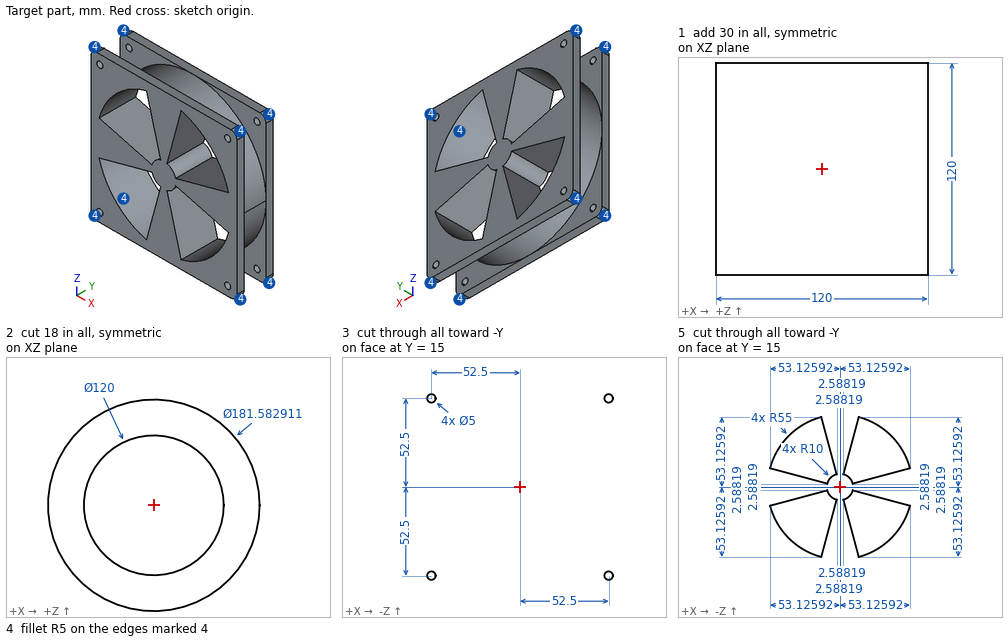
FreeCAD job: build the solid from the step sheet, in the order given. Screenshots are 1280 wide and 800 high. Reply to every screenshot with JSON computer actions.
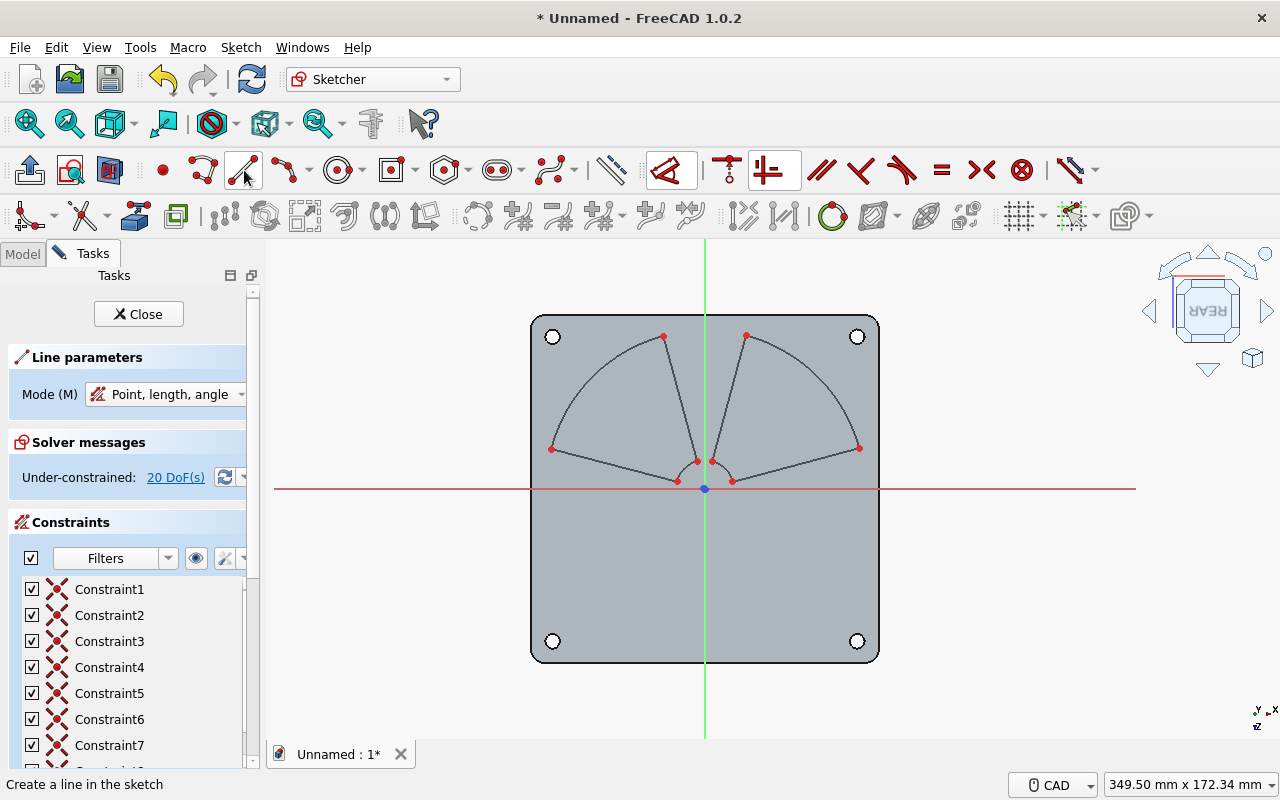
{"action": "scroll", "coordinate": [712, 517], "scroll_direction": "up", "scroll_amount": 4}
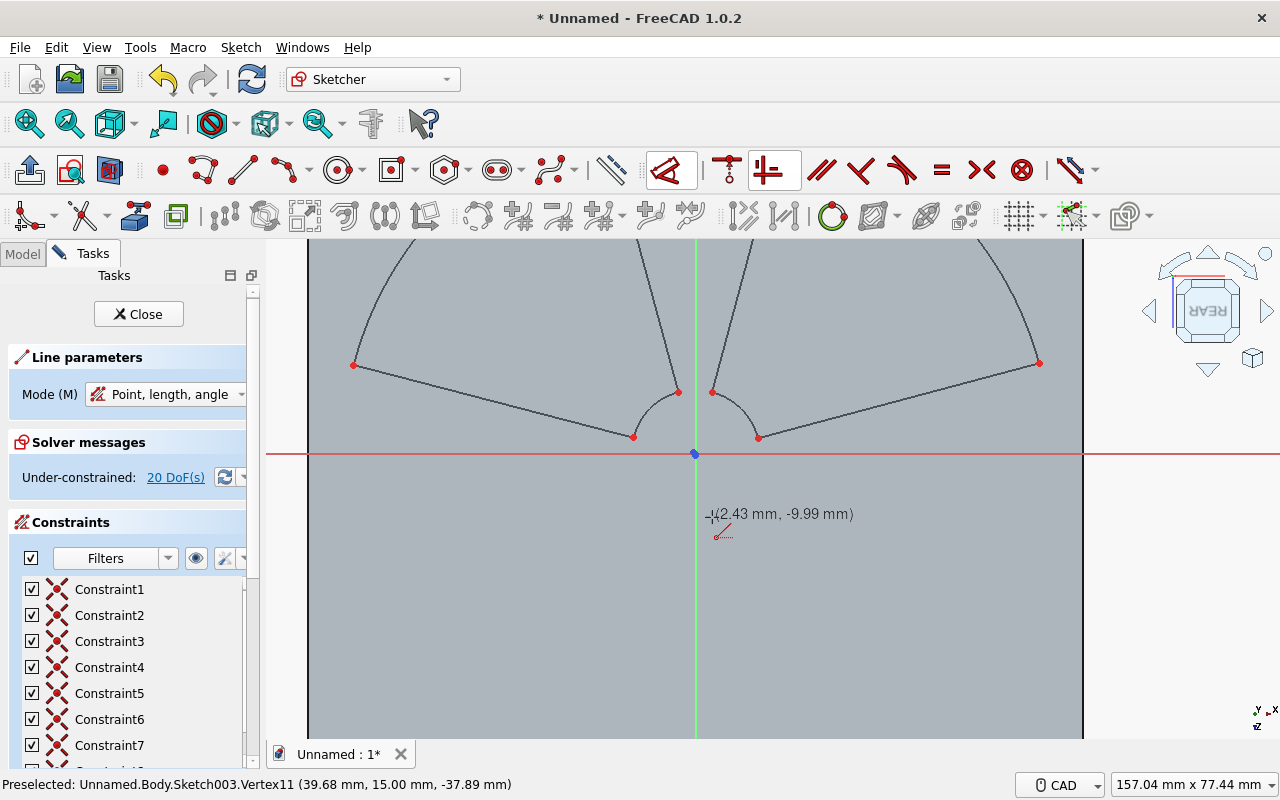
{"action": "left_click", "coordinate": [712, 516]}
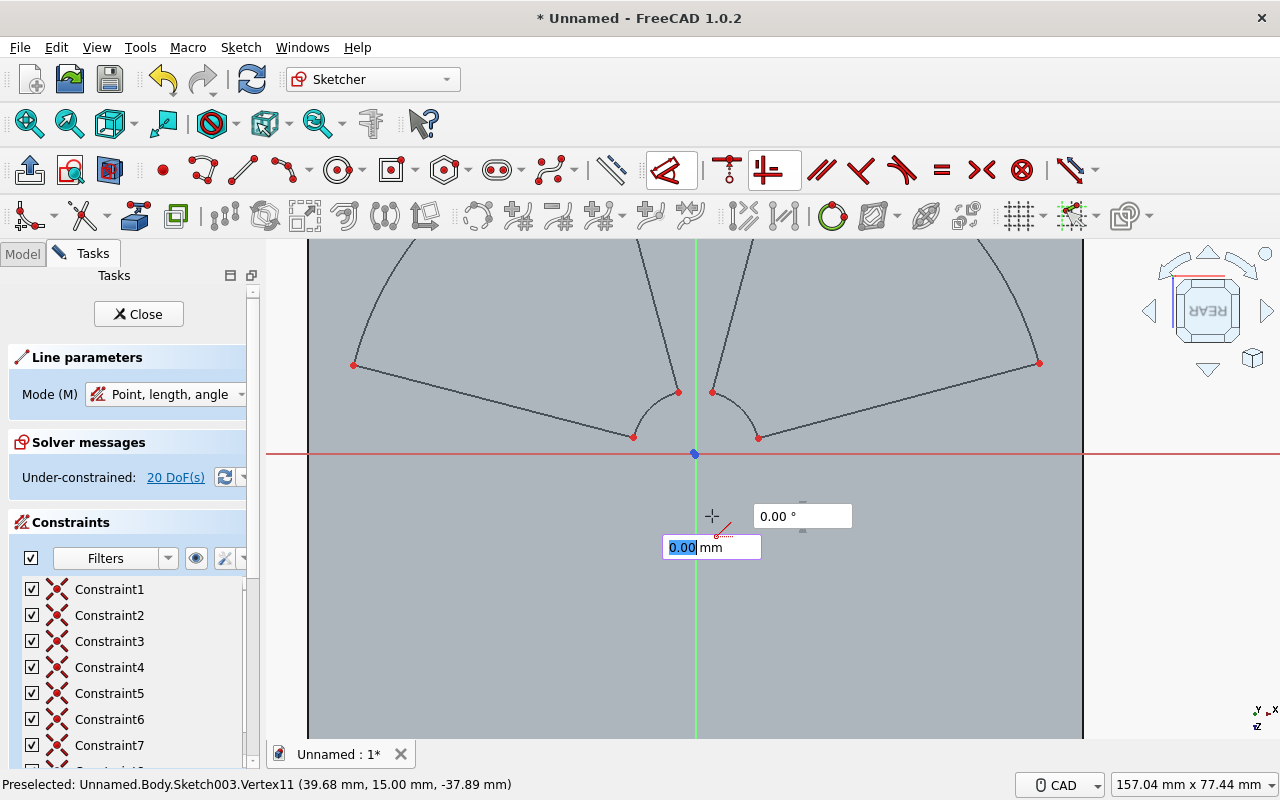
{"action": "scroll", "coordinate": [712, 518], "scroll_direction": "down", "scroll_amount": 4}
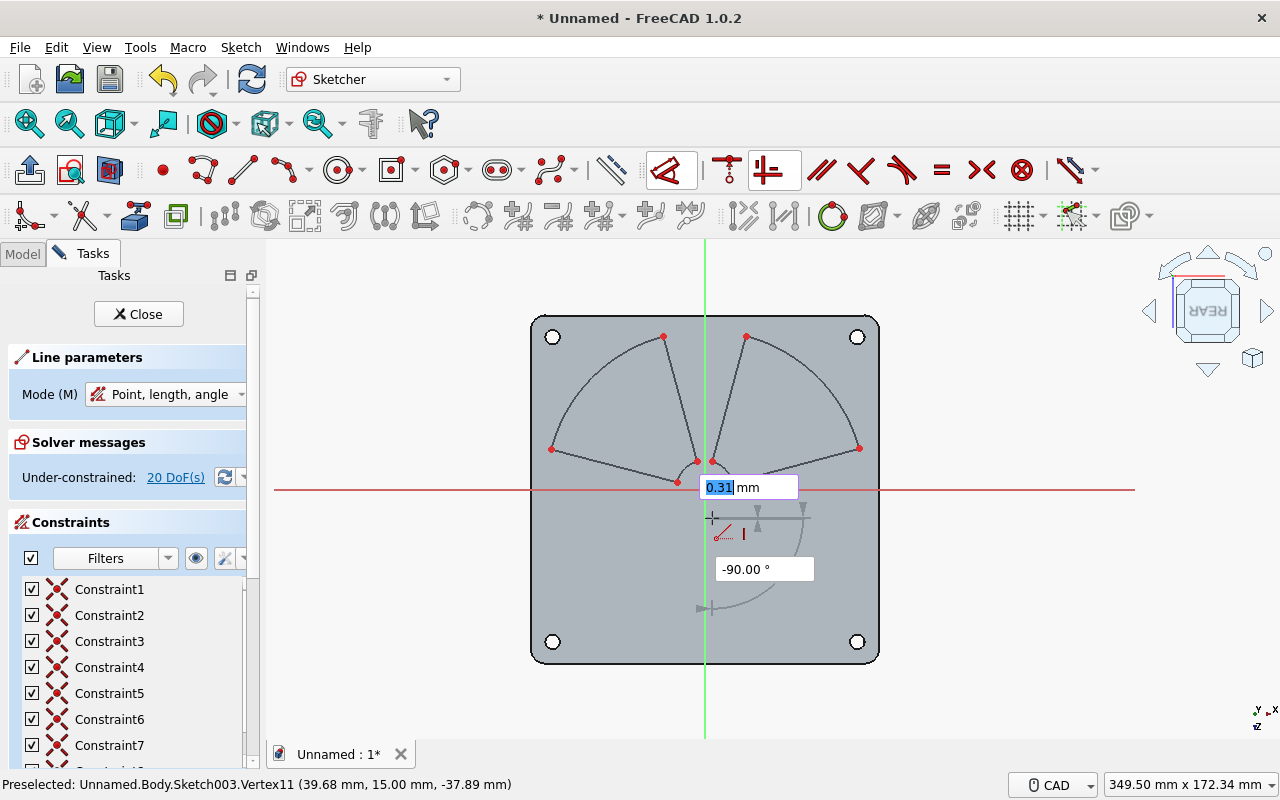
{"action": "left_click", "coordinate": [746, 644]}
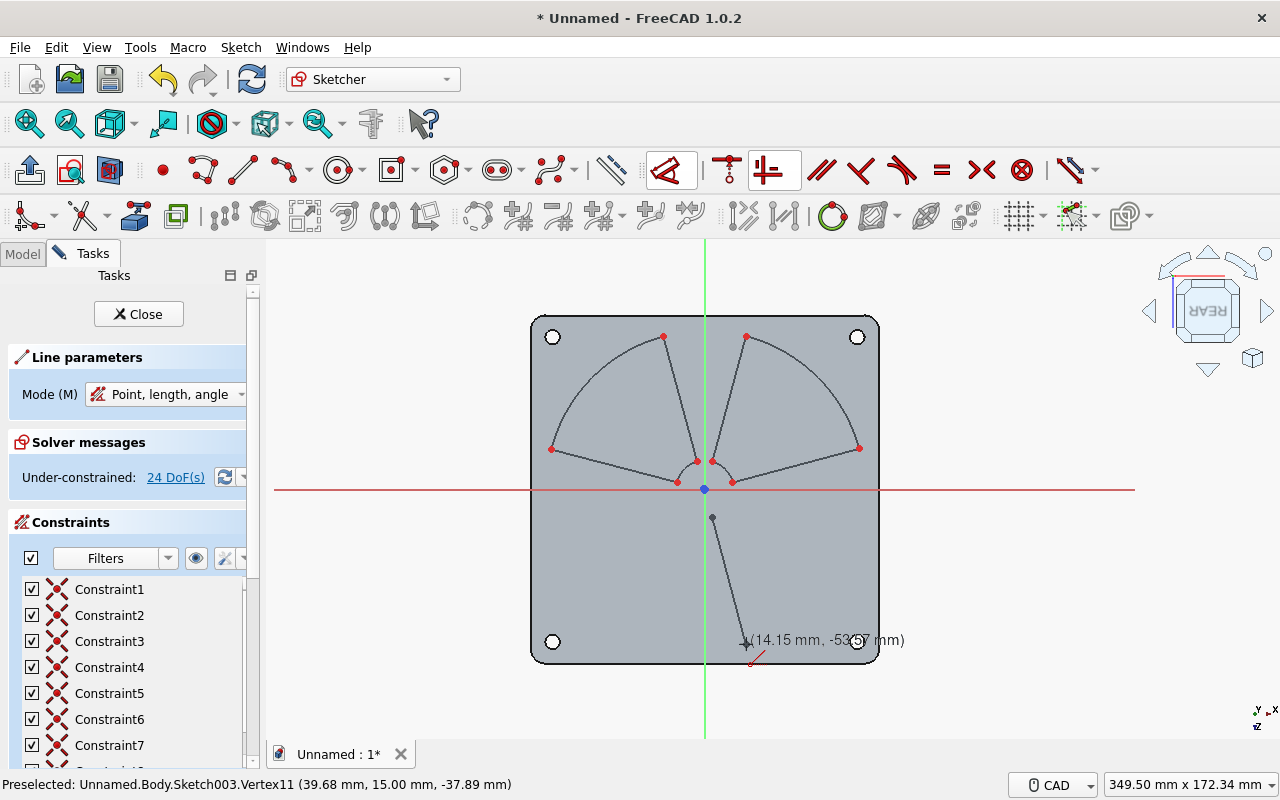
{"action": "left_click", "coordinate": [859, 531]}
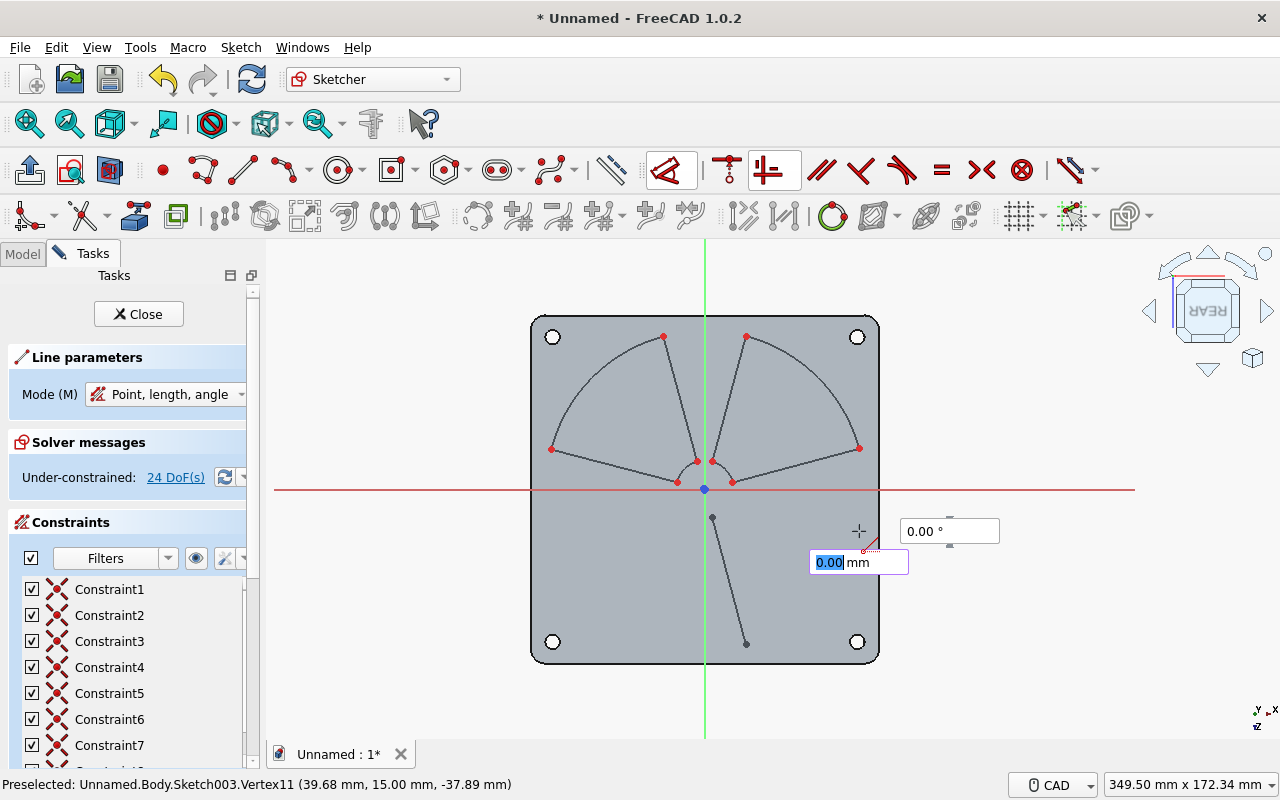
{"action": "scroll", "coordinate": [733, 497], "scroll_direction": "up", "scroll_amount": 4}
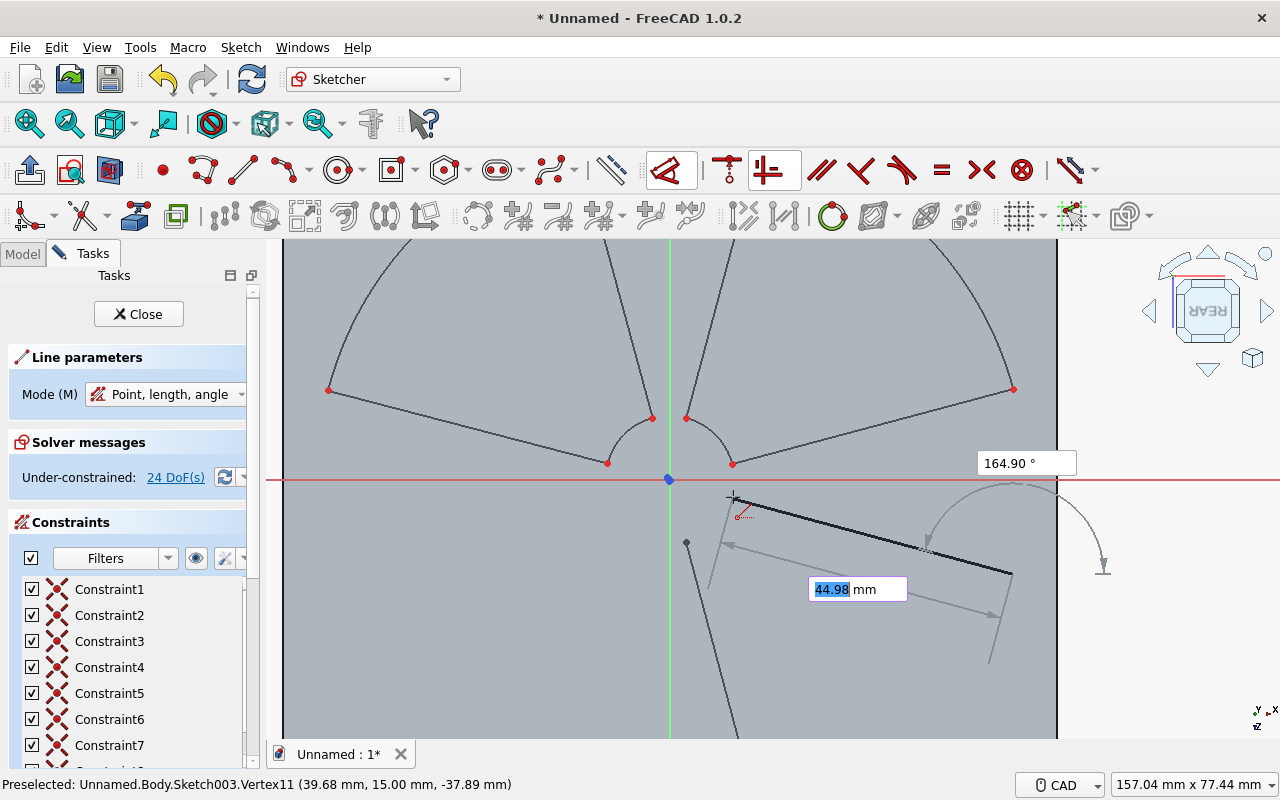
{"action": "left_click", "coordinate": [732, 497]}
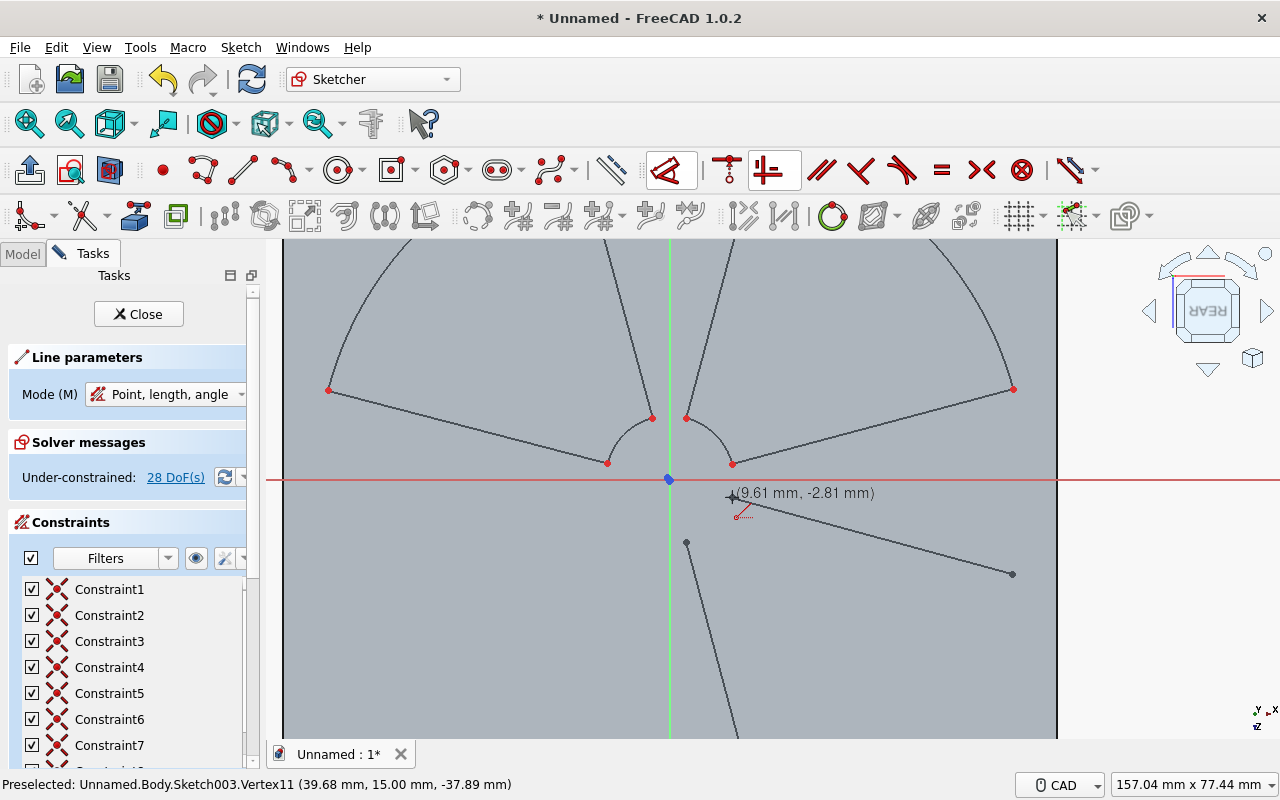
{"action": "left_click", "coordinate": [284, 170]}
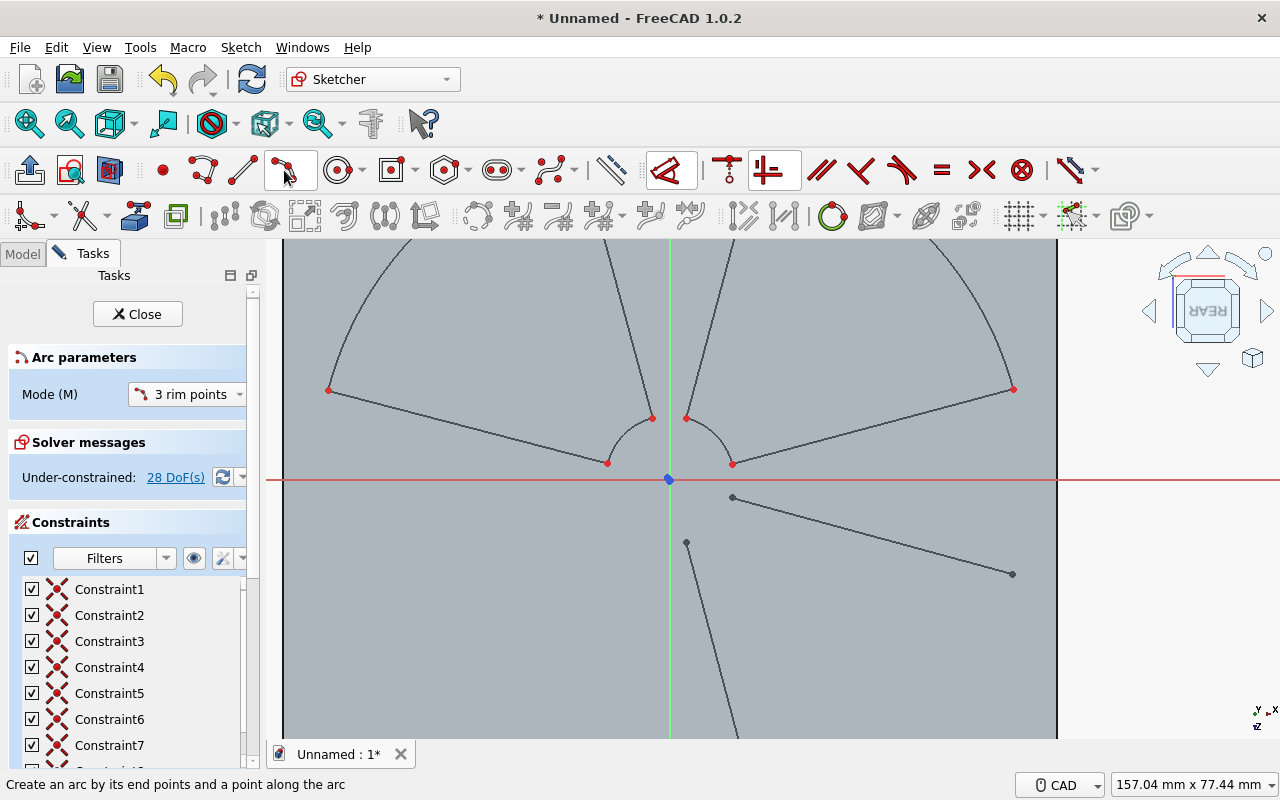
{"action": "scroll", "coordinate": [733, 496], "scroll_direction": "down", "scroll_amount": 4}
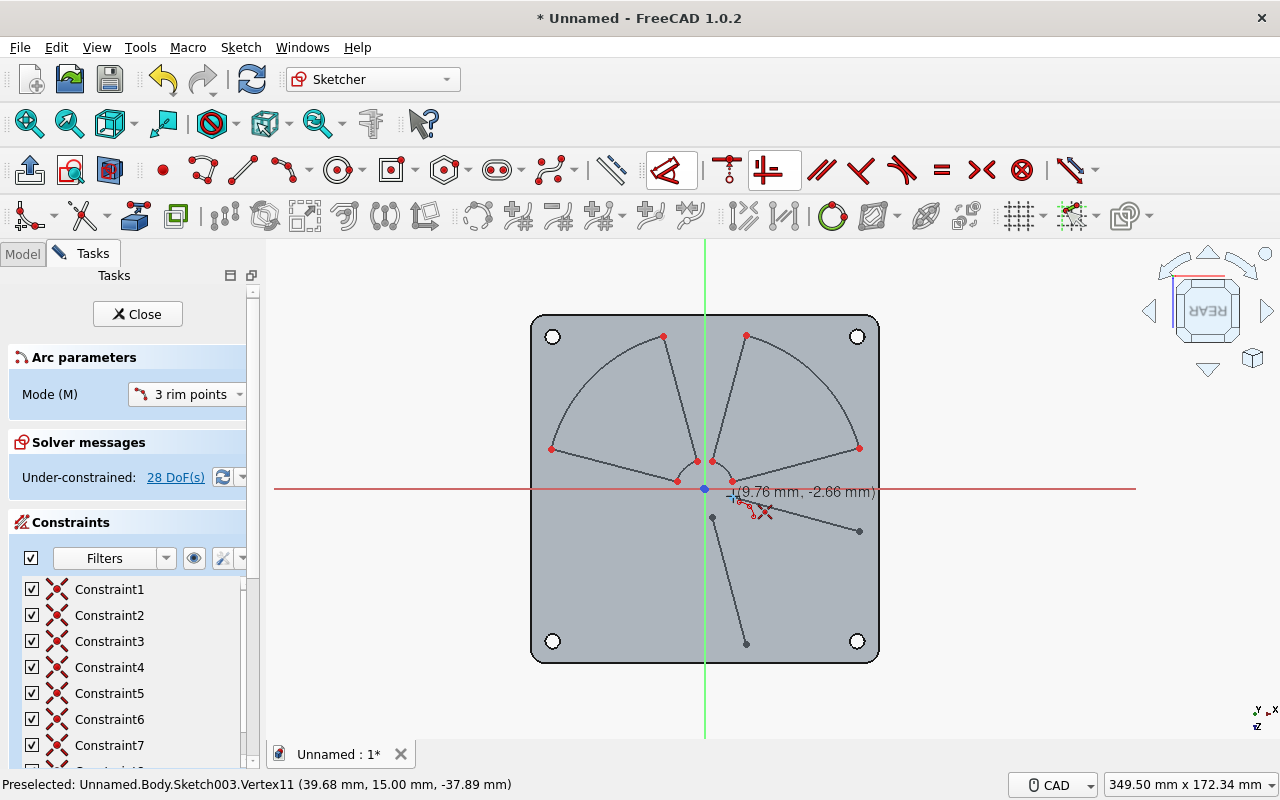
{"action": "left_click", "coordinate": [746, 644]}
{"action": "left_click", "coordinate": [859, 531]}
{"action": "left_click", "coordinate": [818, 602]}